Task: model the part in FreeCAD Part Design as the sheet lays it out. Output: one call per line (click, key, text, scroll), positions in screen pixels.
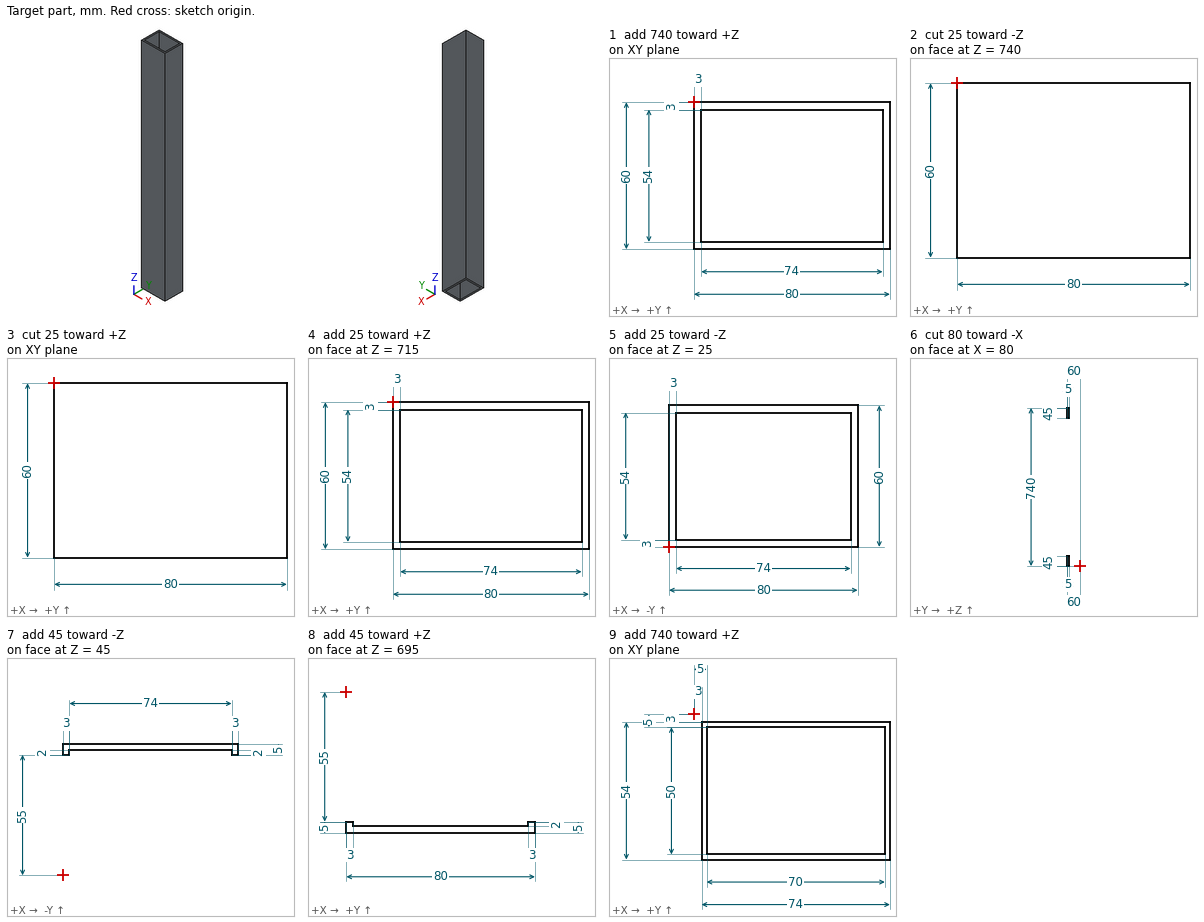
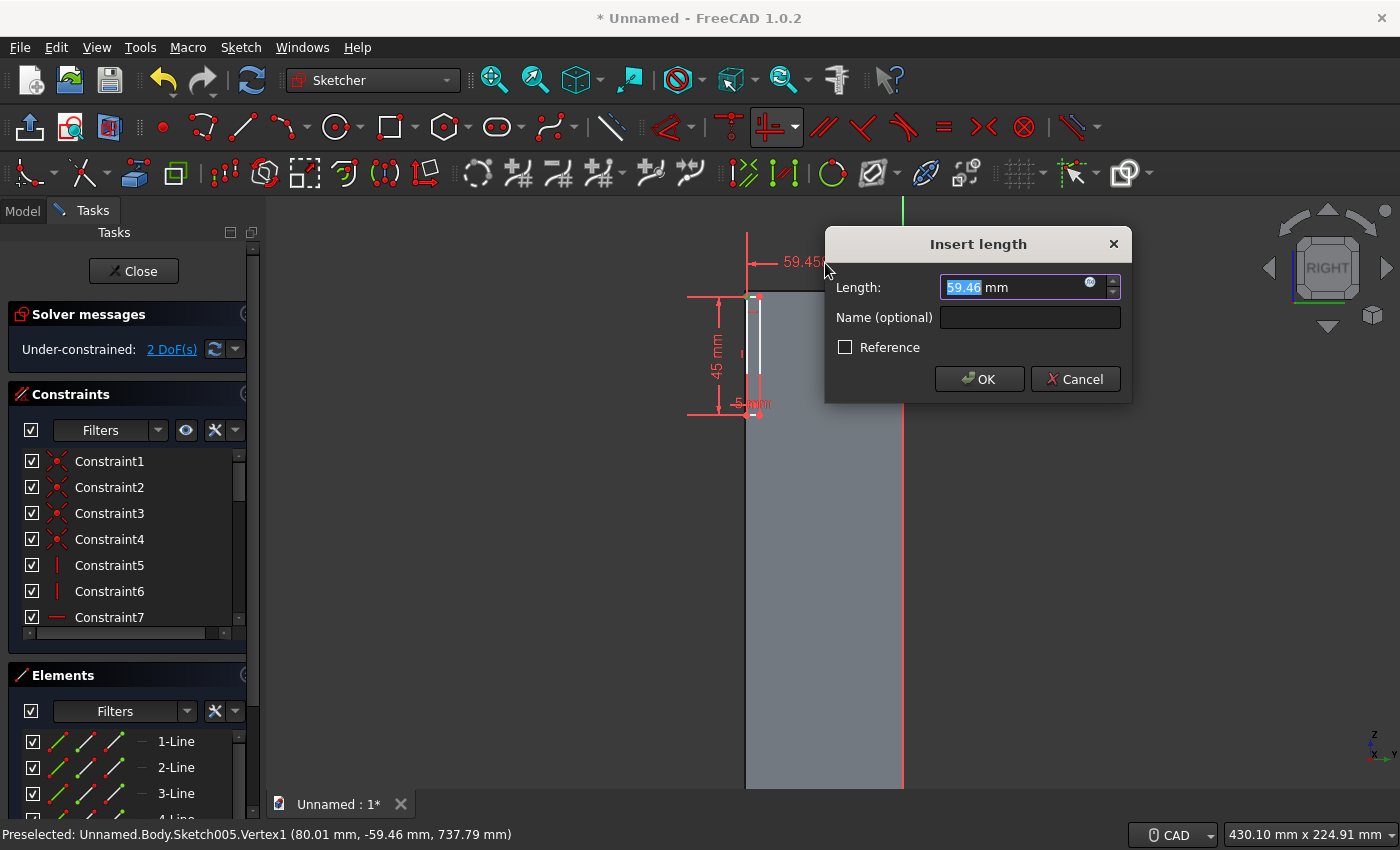
text(60)
key(Return)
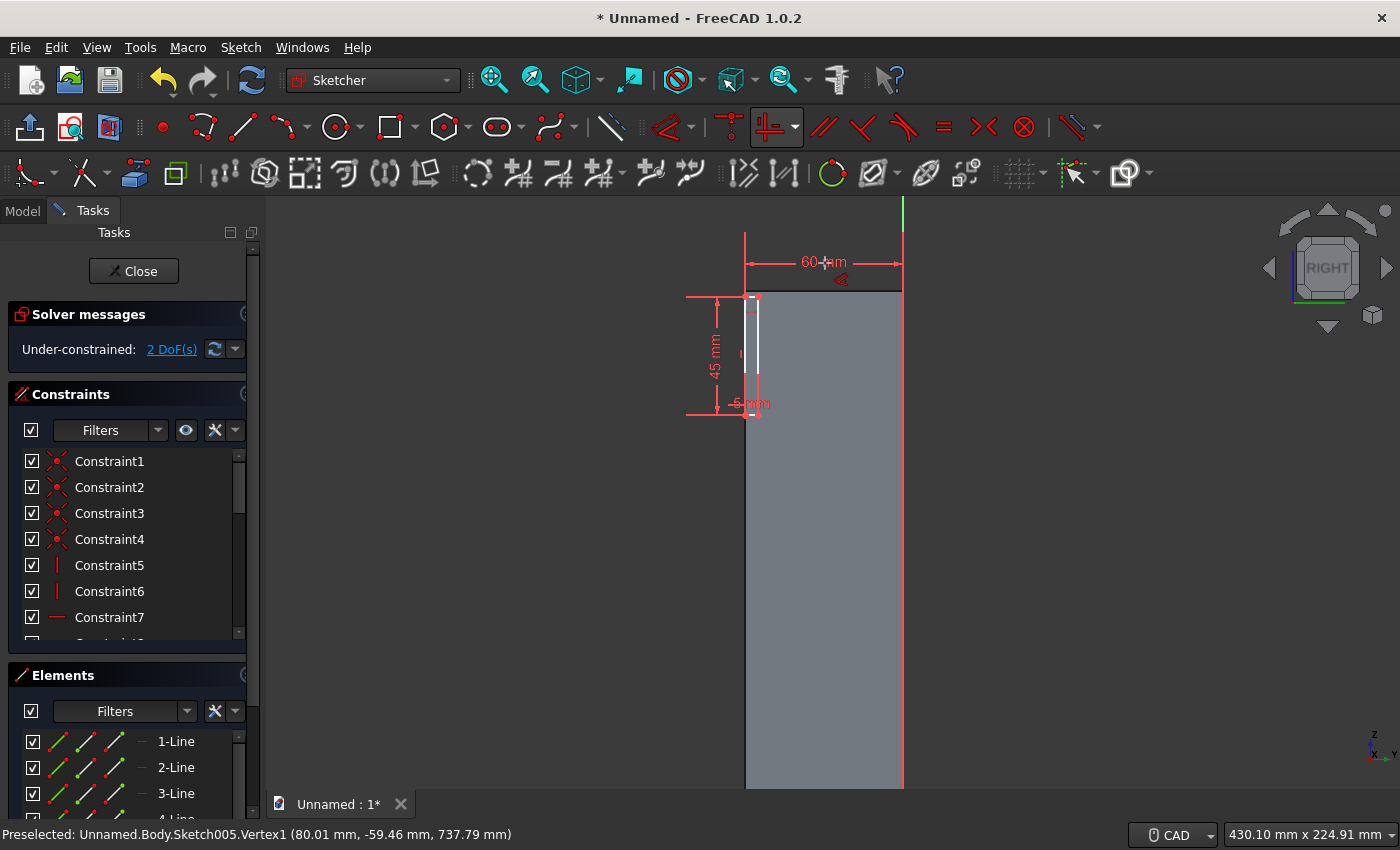
scroll(749, 297, down, 8)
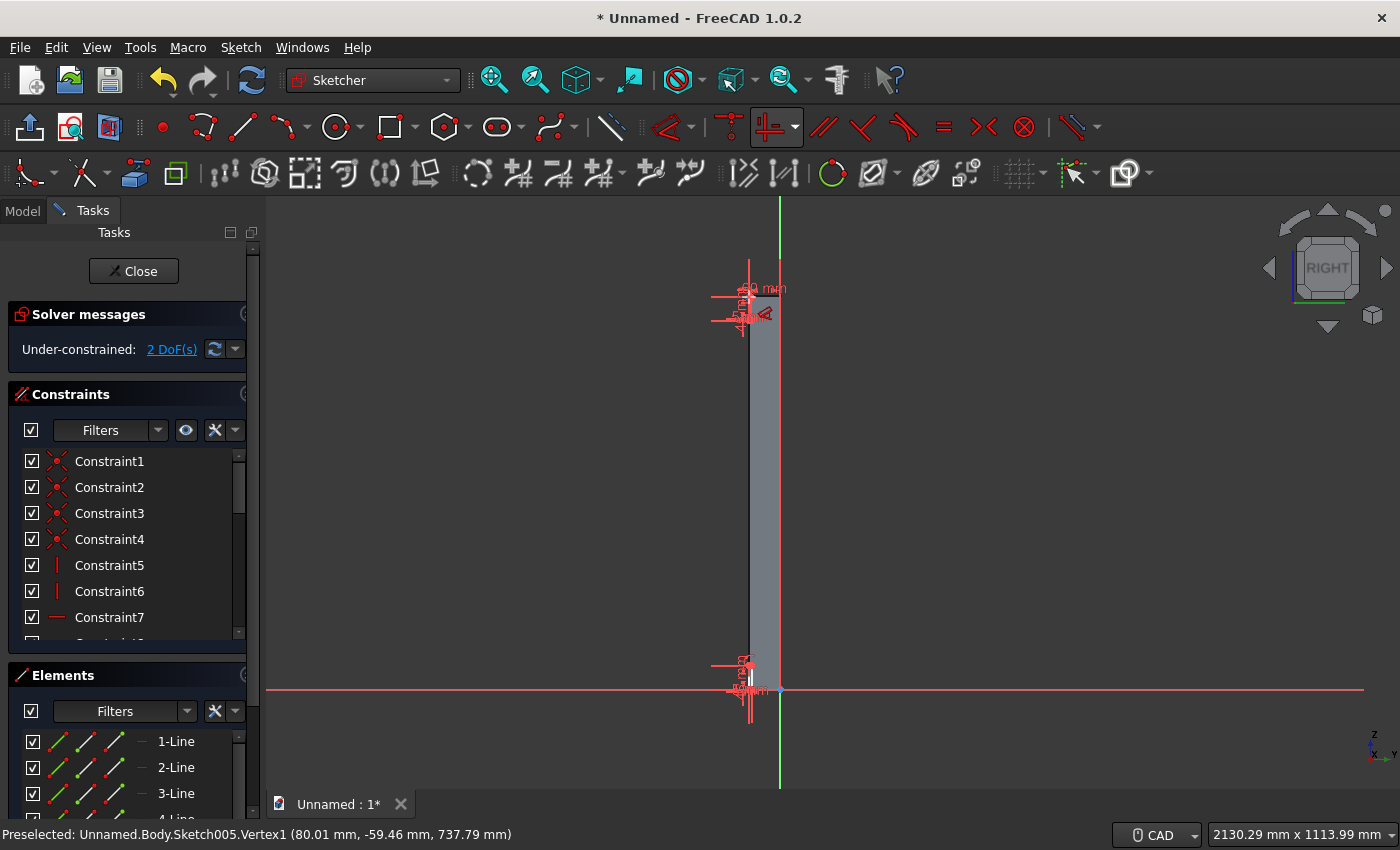
scroll(749, 666, up, 8)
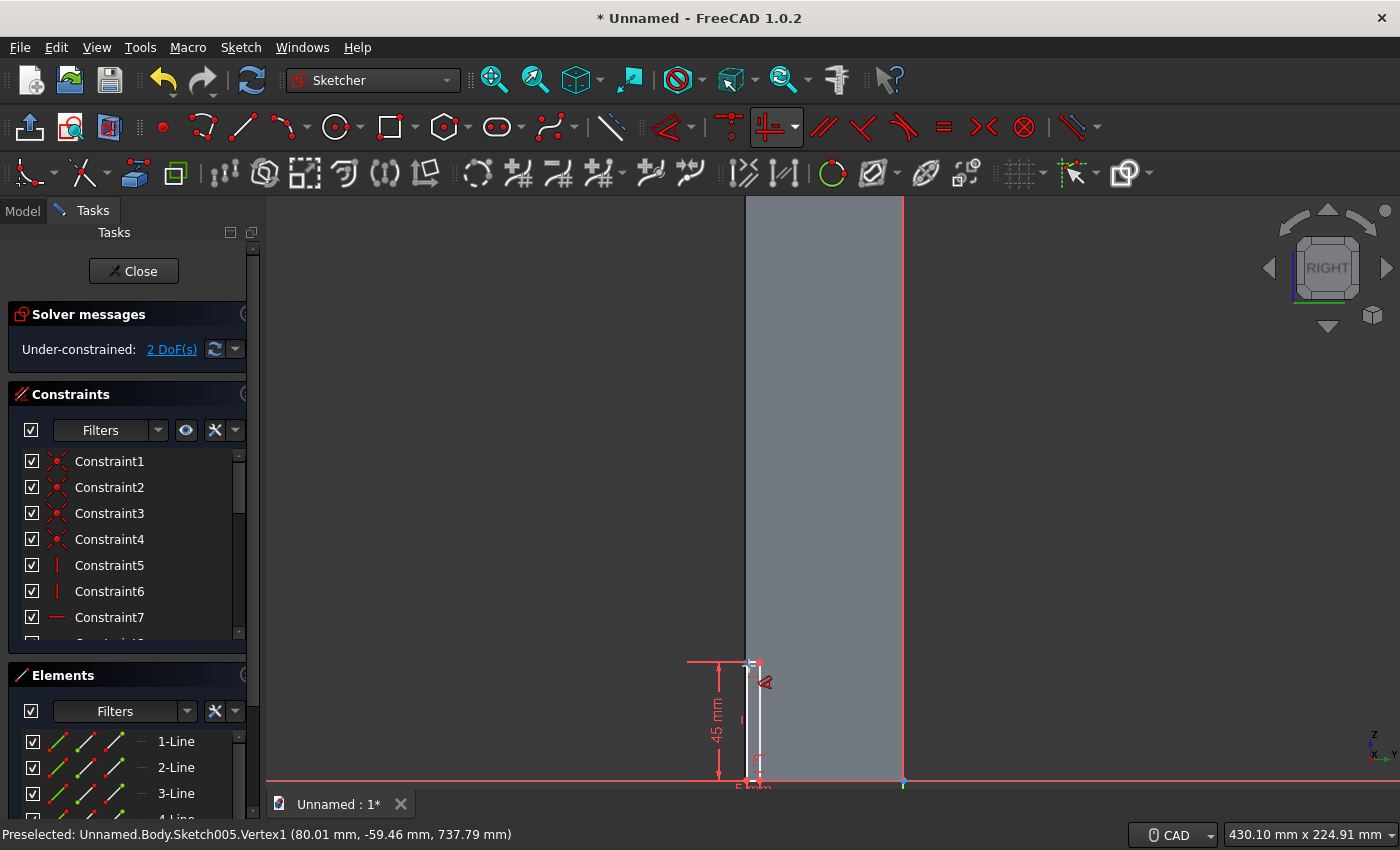
click(747, 662)
click(825, 628)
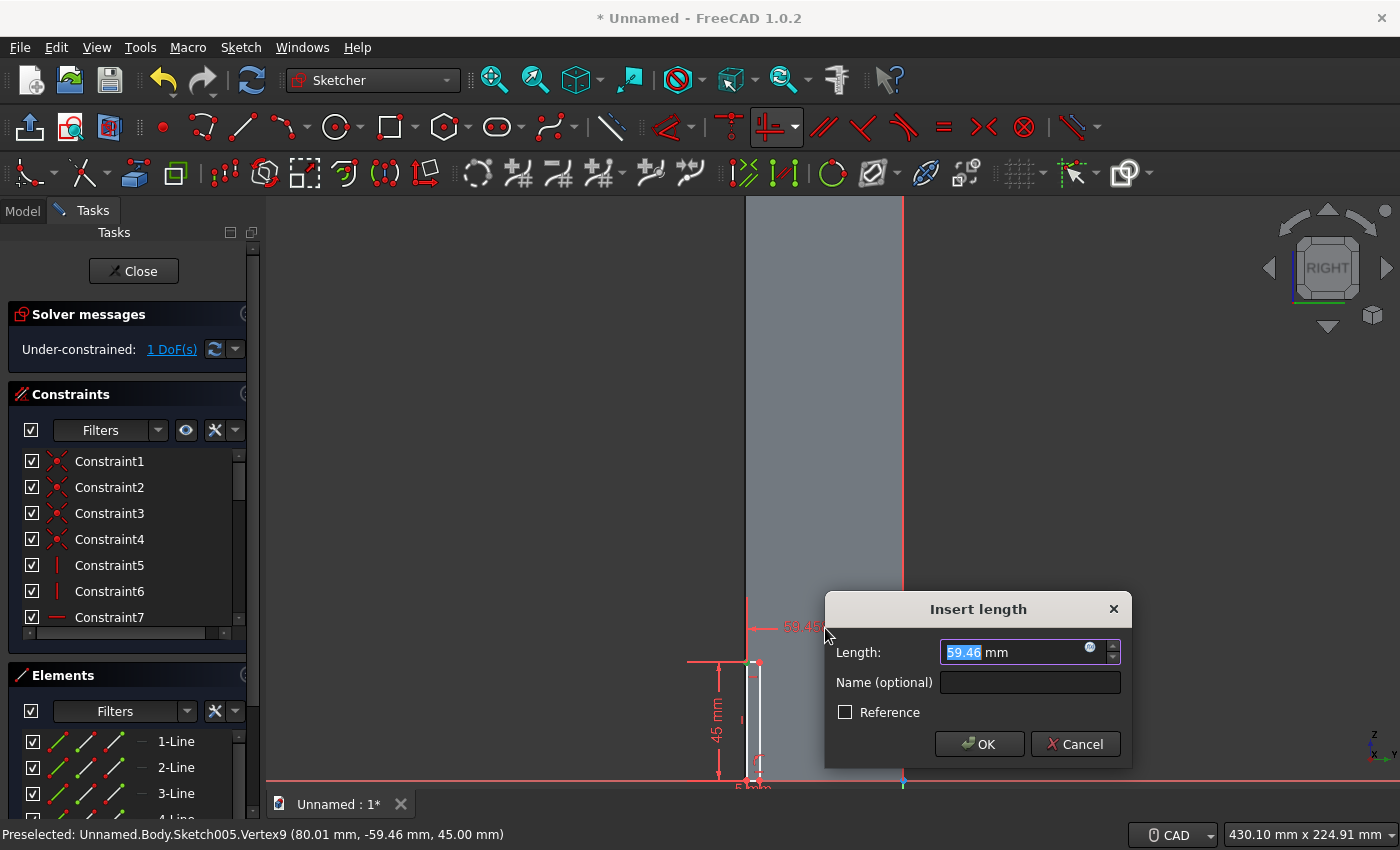
text(60)
key(Return)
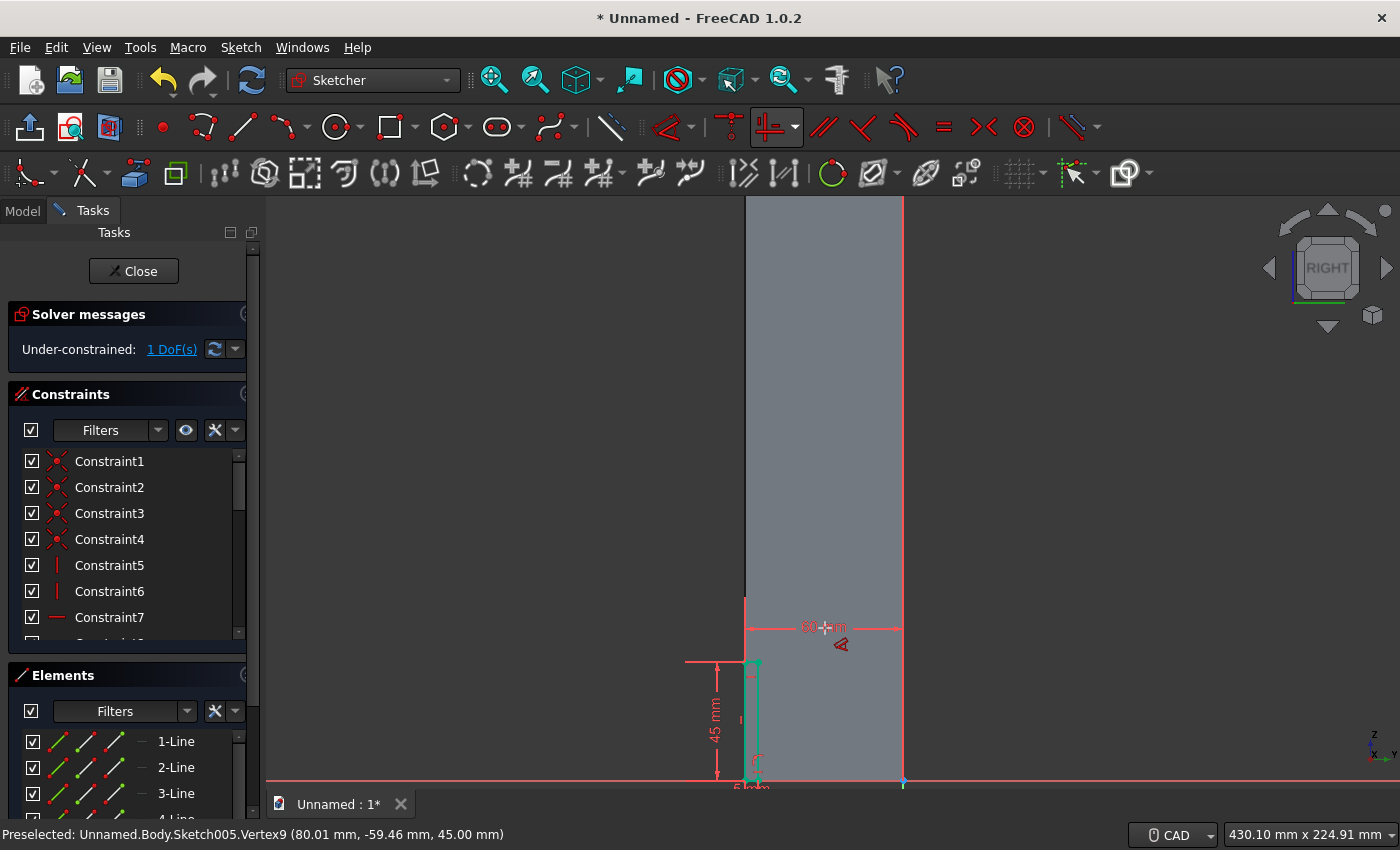
scroll(749, 666, down, 8)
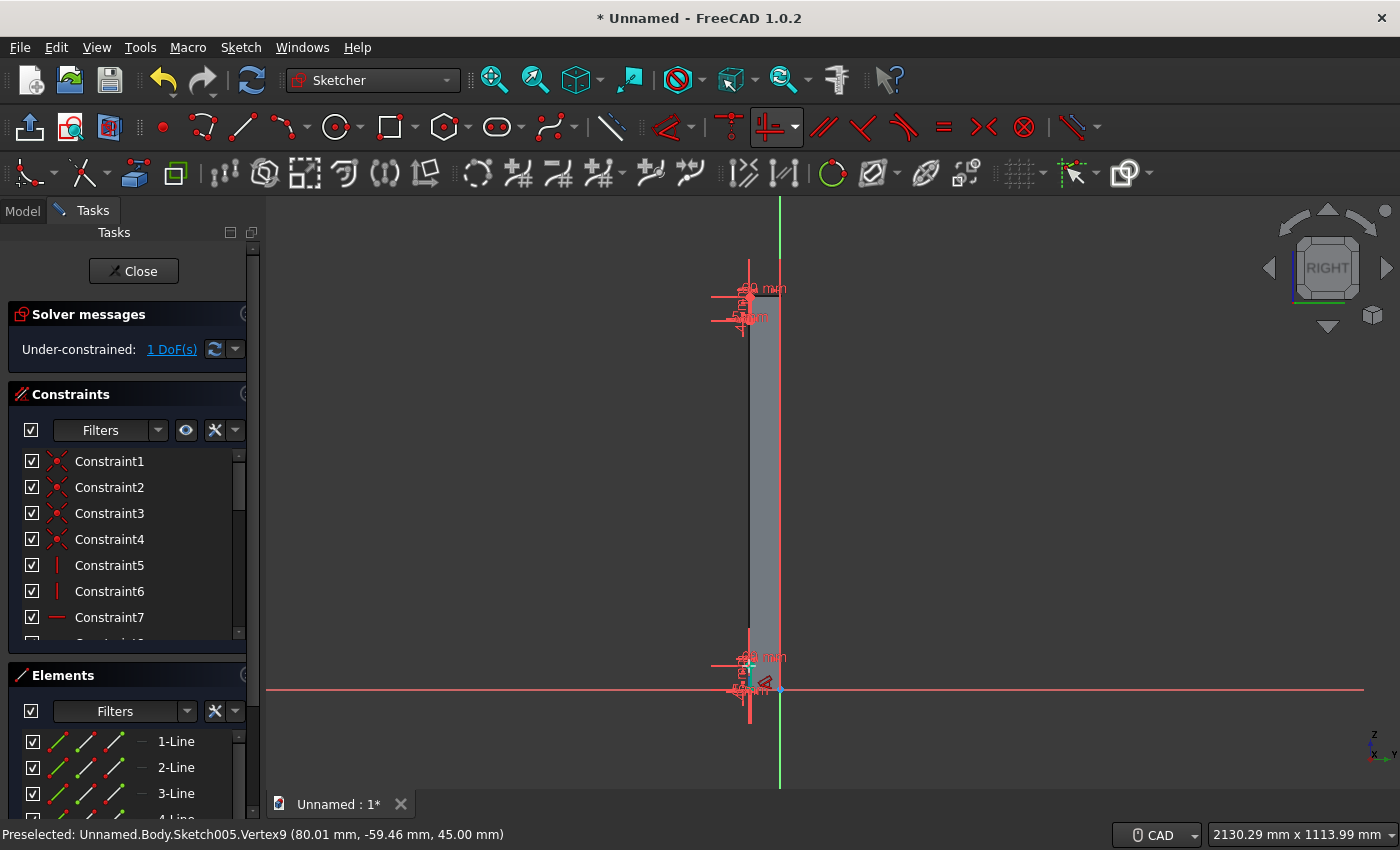
scroll(749, 297, up, 8)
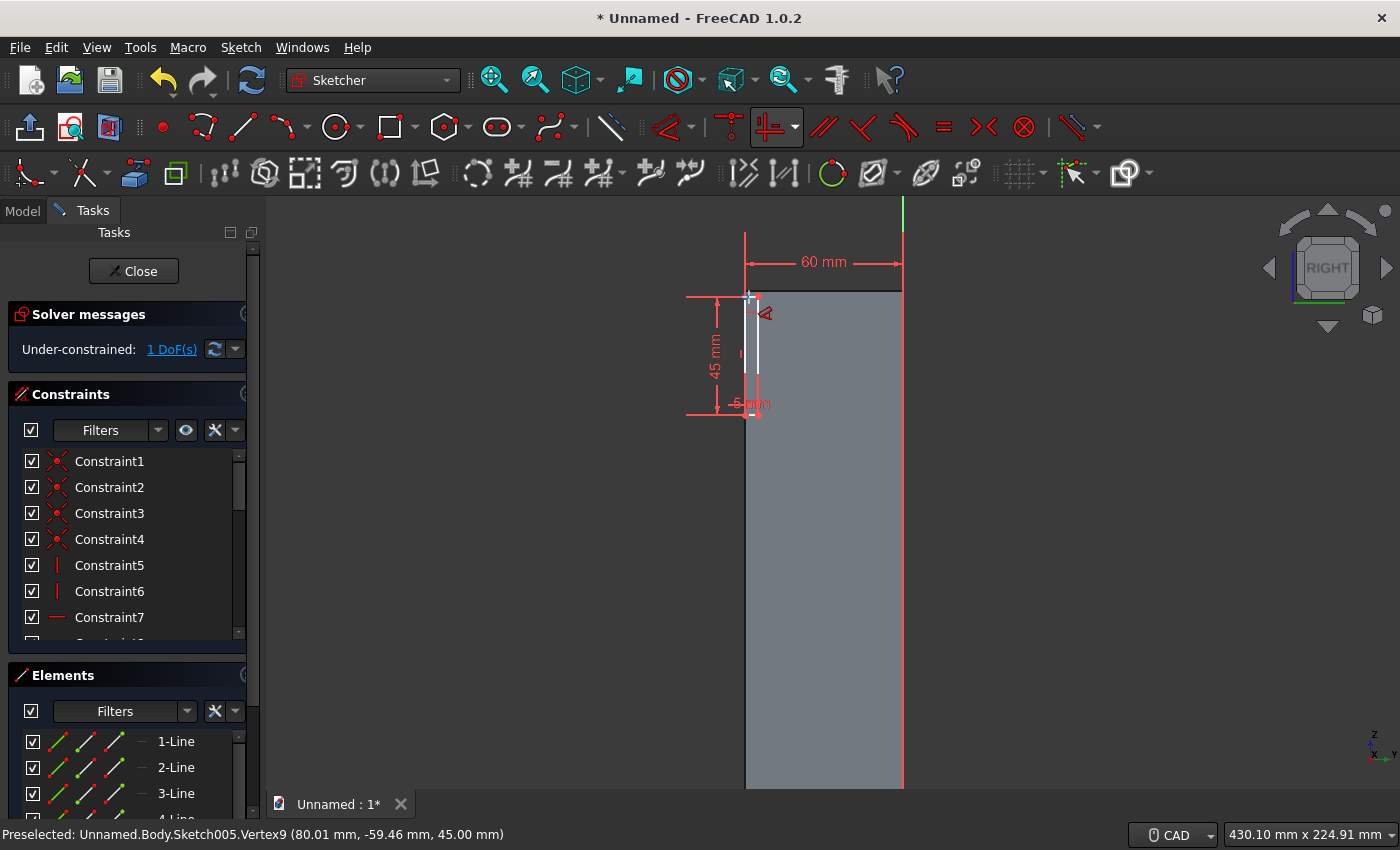
click(745, 297)
click(937, 529)